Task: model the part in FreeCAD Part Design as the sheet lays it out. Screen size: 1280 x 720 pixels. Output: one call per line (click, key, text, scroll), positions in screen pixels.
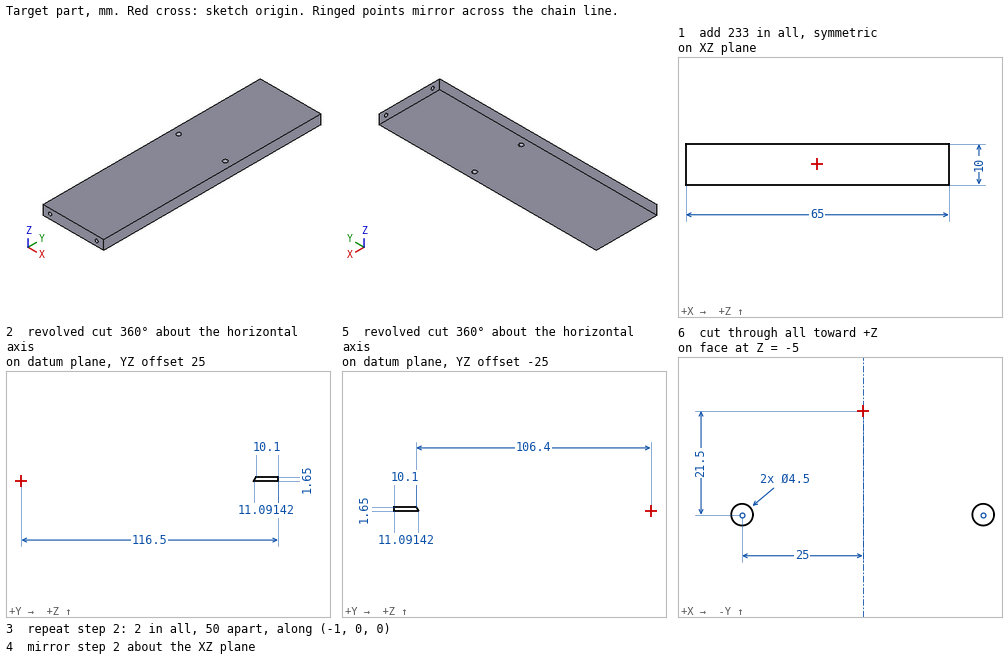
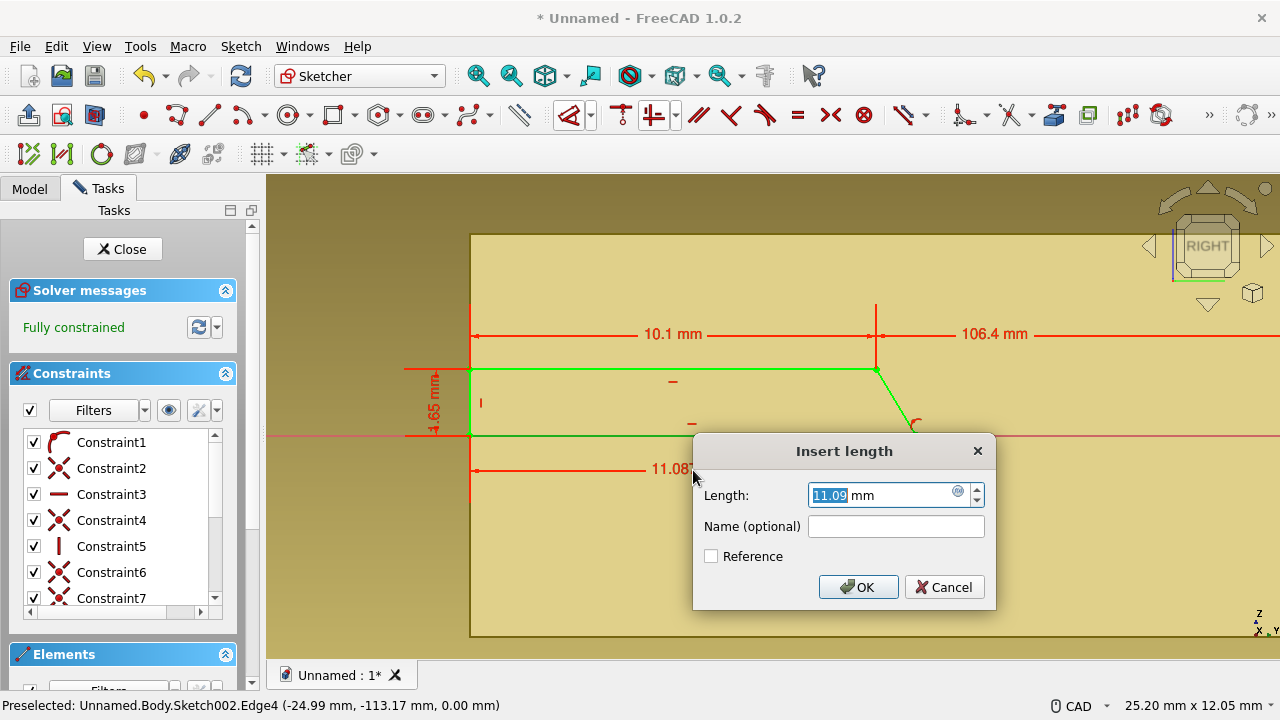
text(11.09142)
key(Return)
key(Escape)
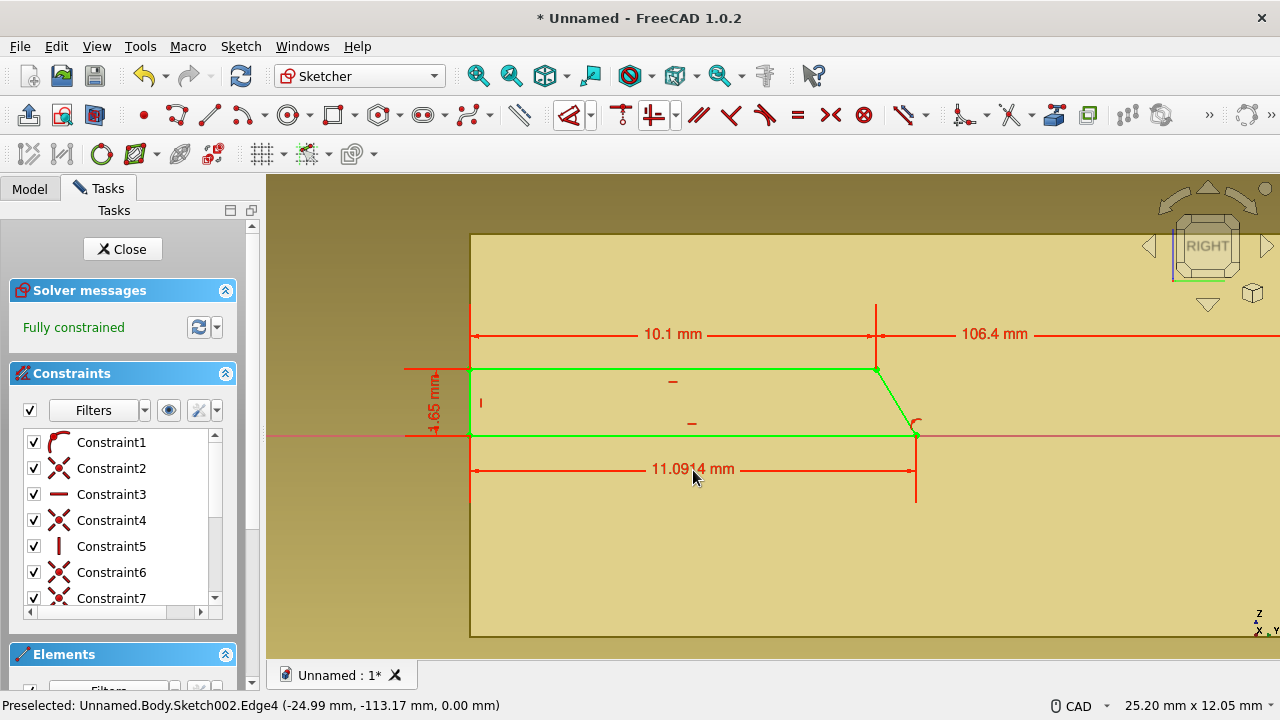
click(123, 249)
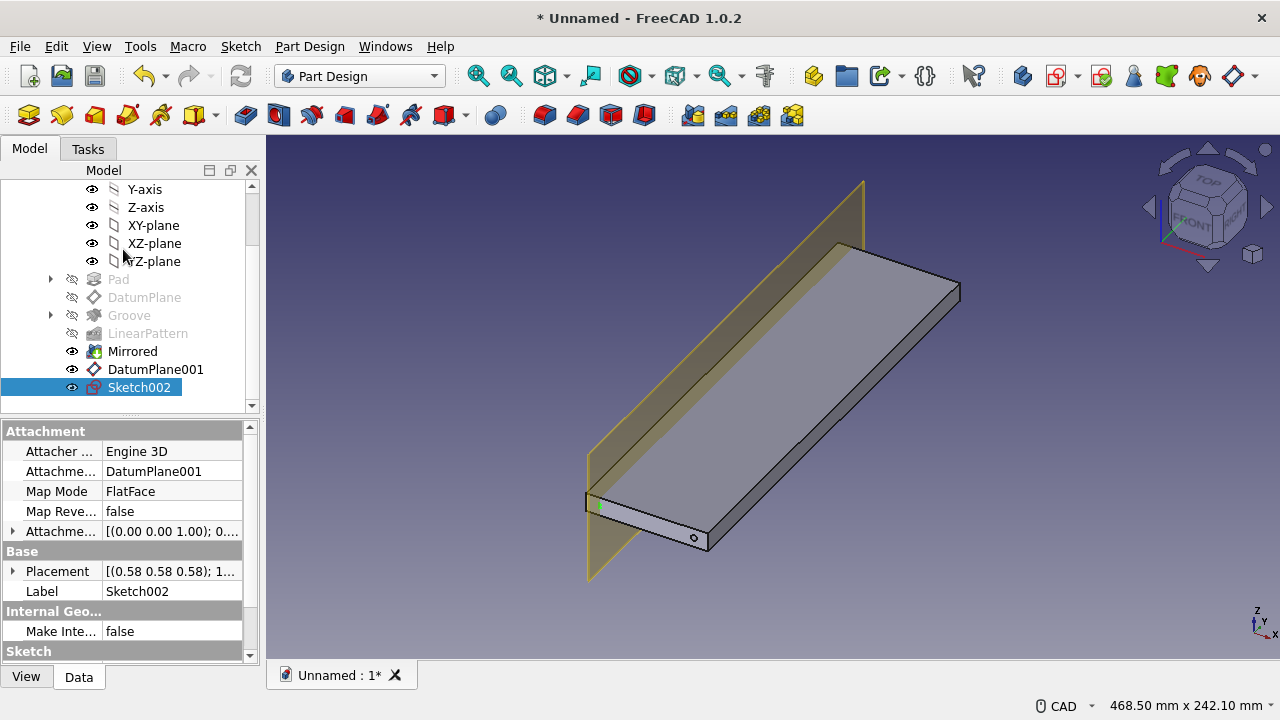
click(312, 116)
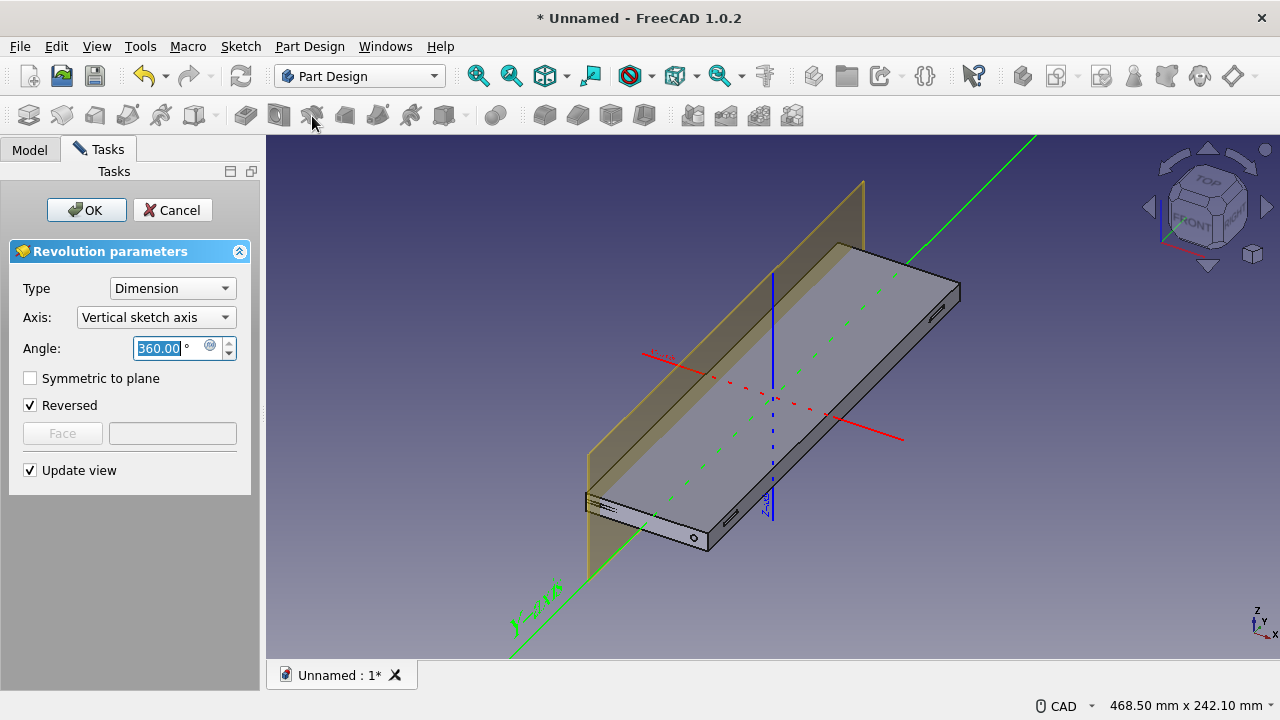
click(157, 318)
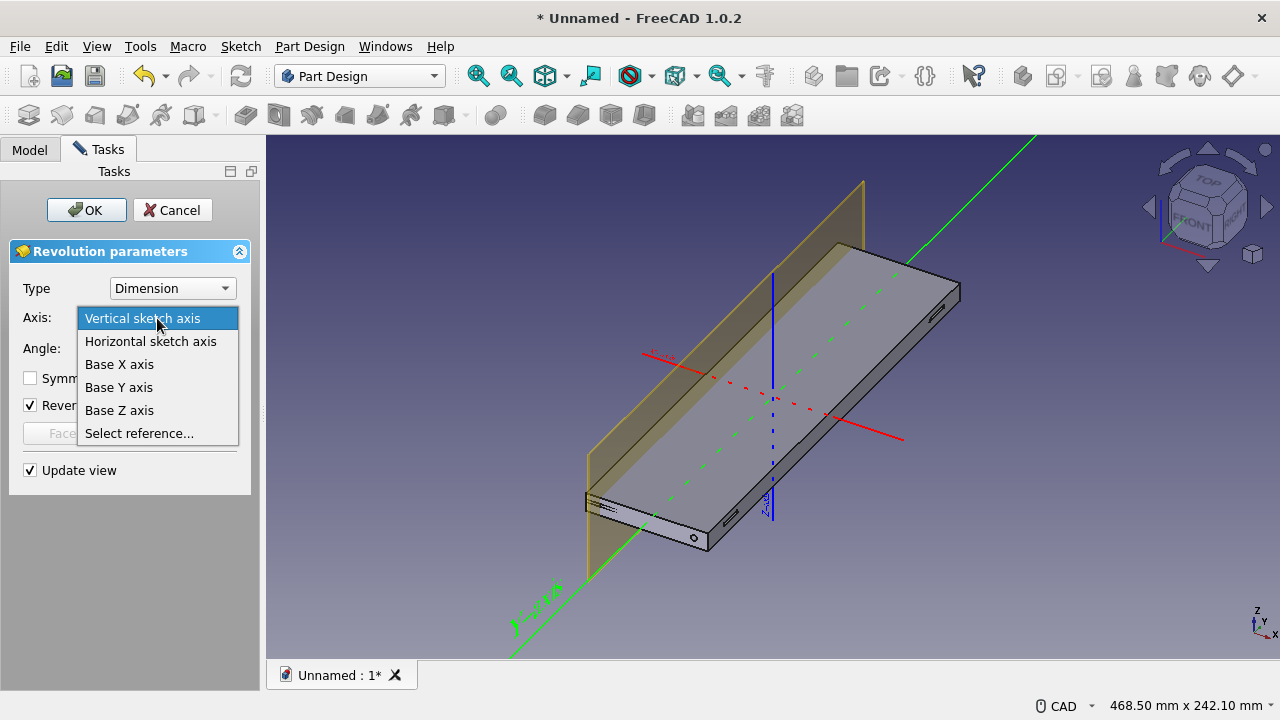
click(156, 342)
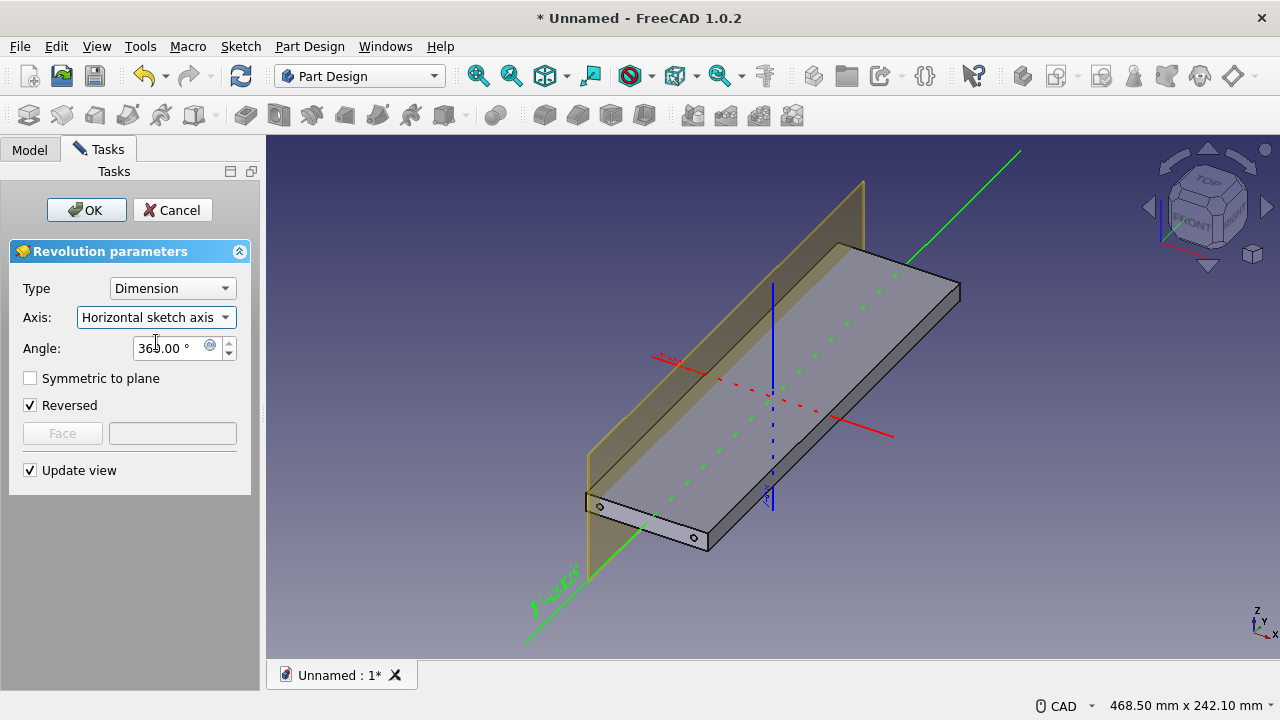
click(87, 210)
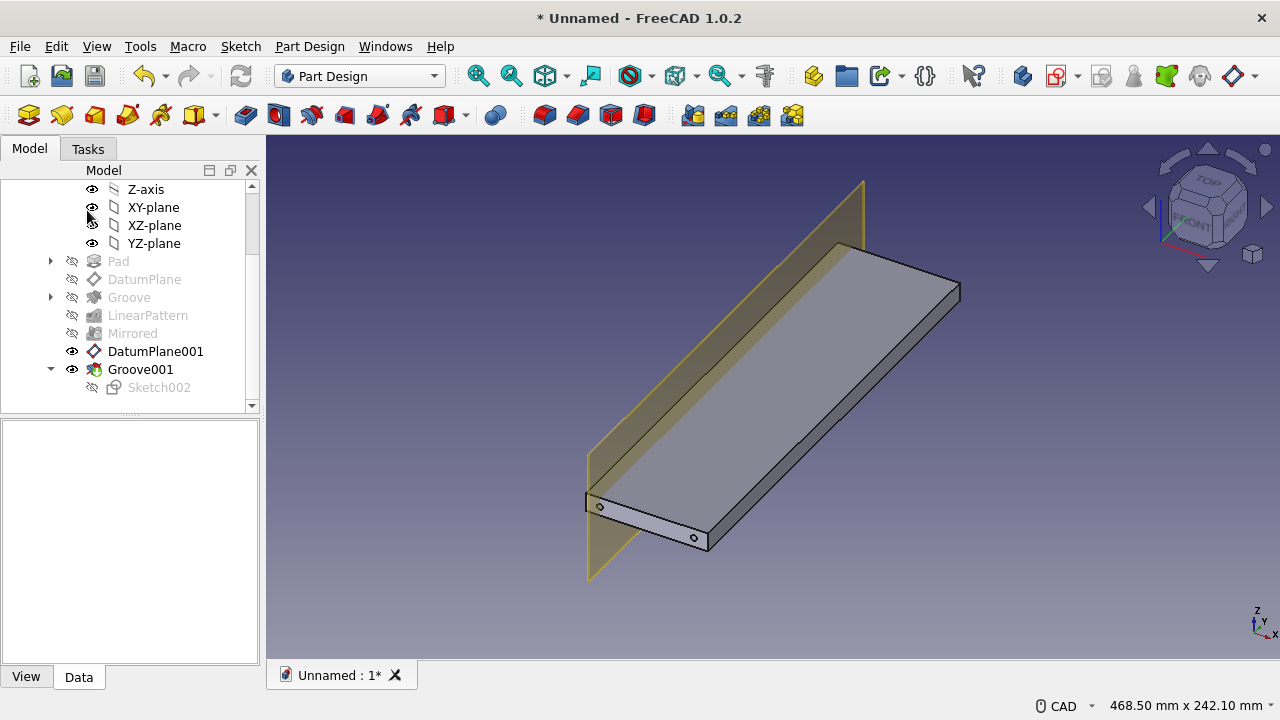
click(117, 351)
key(space)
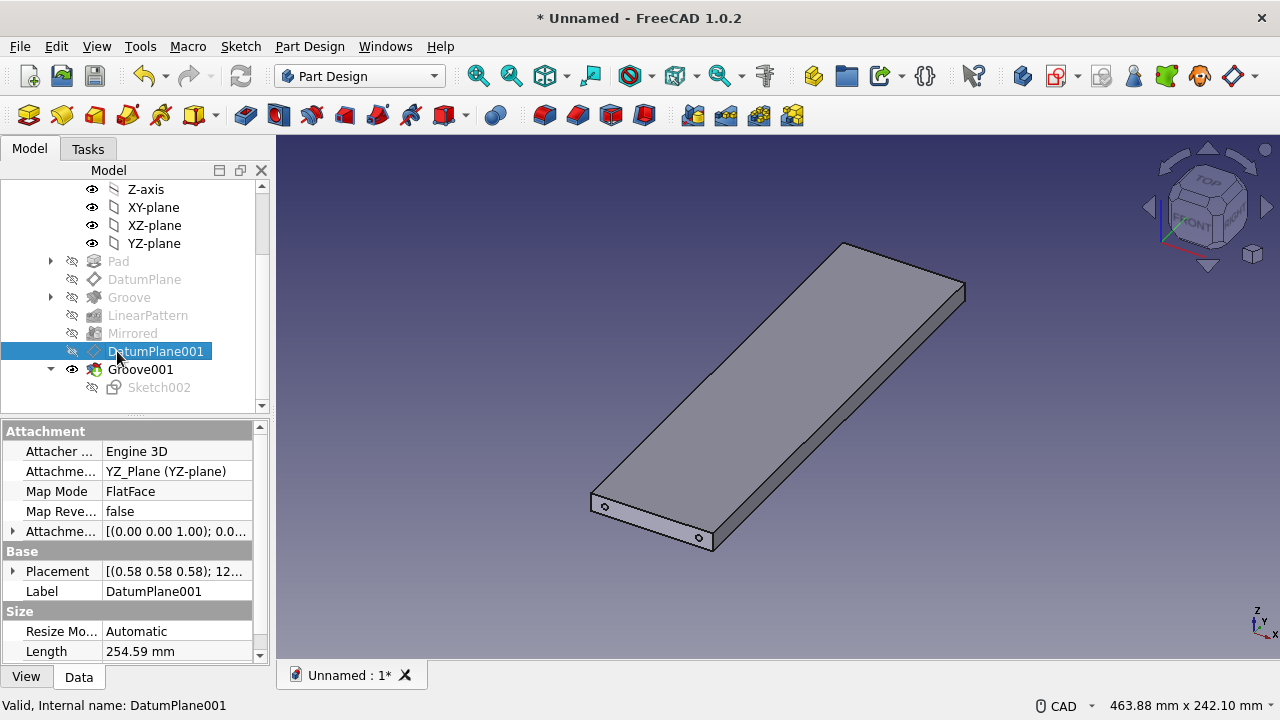
key(5)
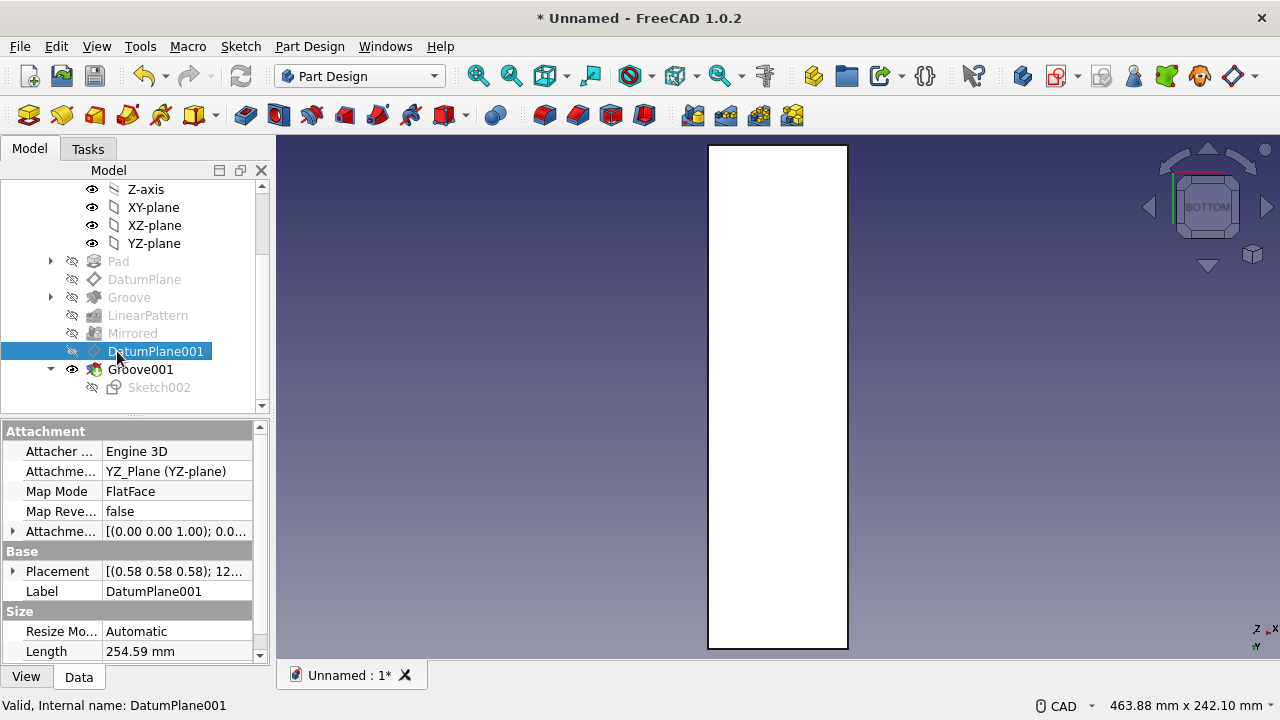
click(778, 540)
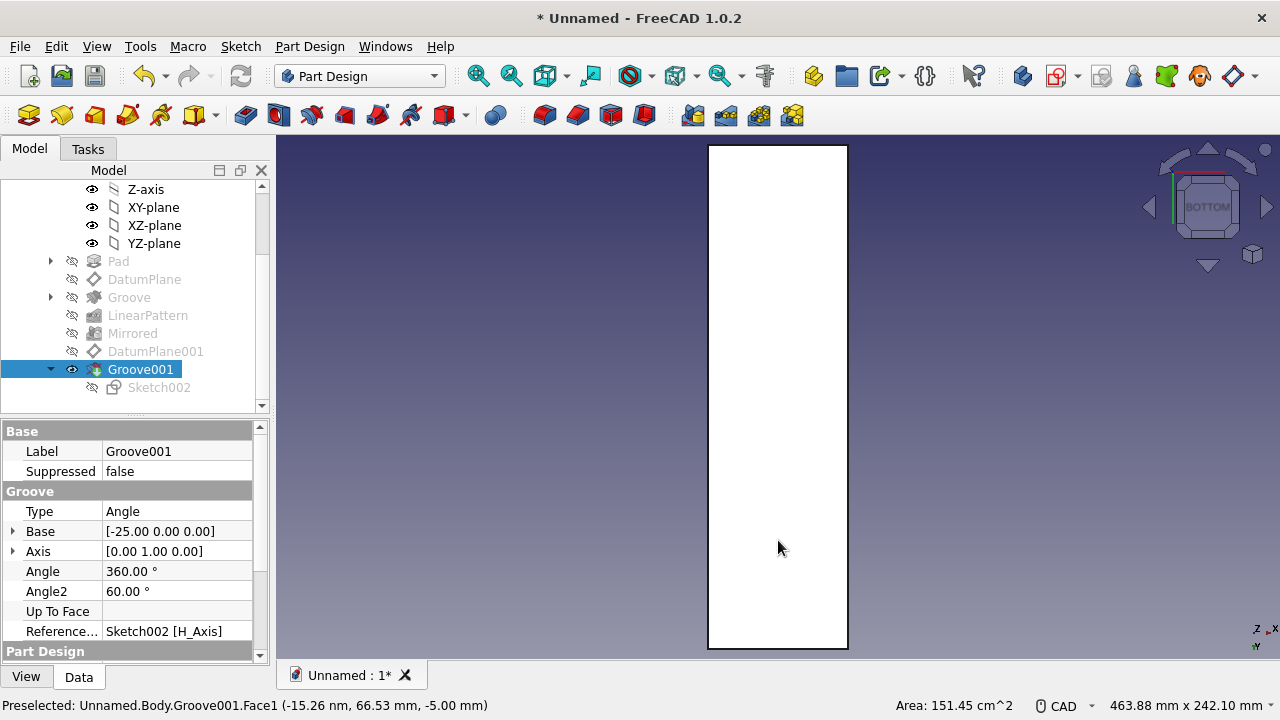
click(1056, 76)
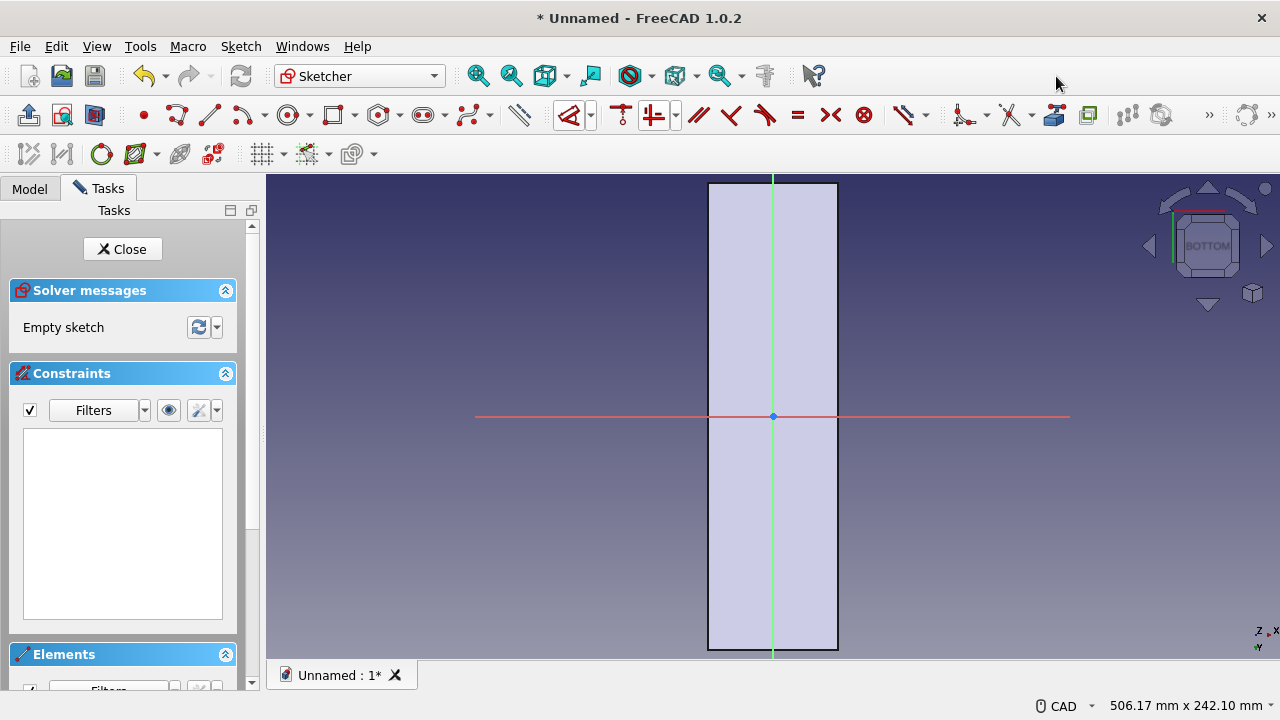
scroll(790, 446, up, 8)